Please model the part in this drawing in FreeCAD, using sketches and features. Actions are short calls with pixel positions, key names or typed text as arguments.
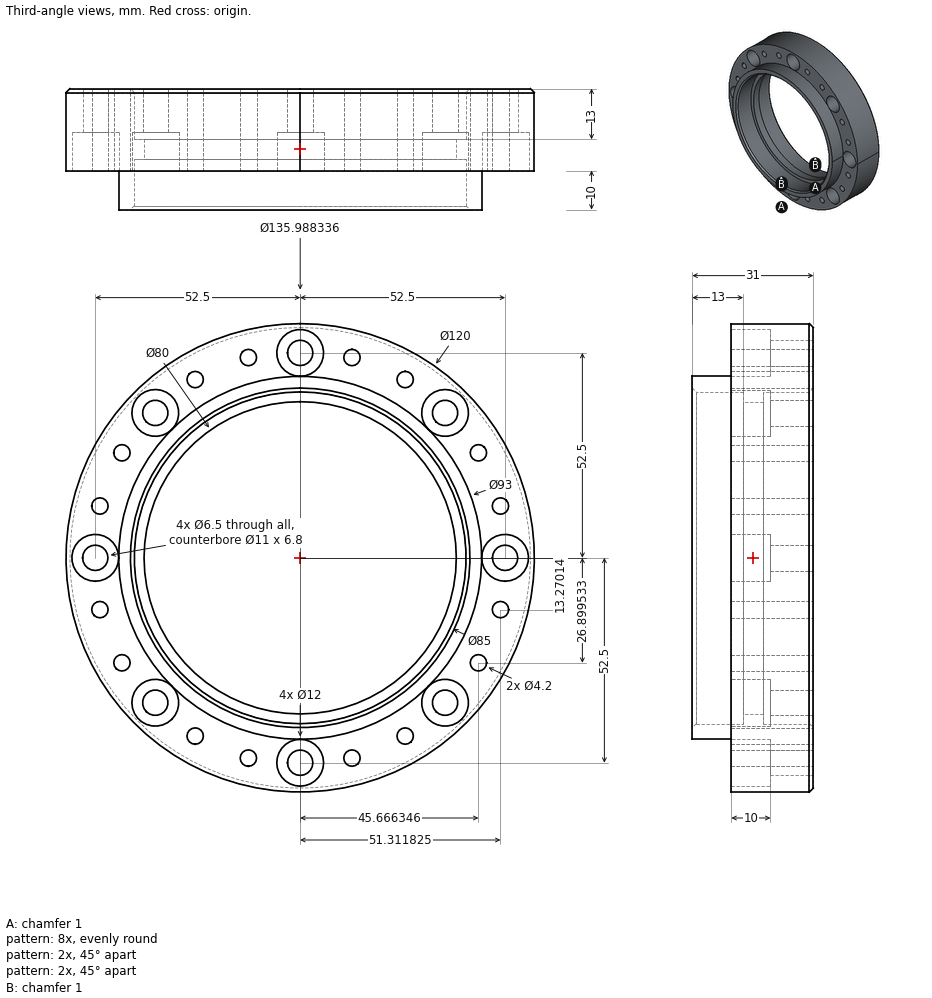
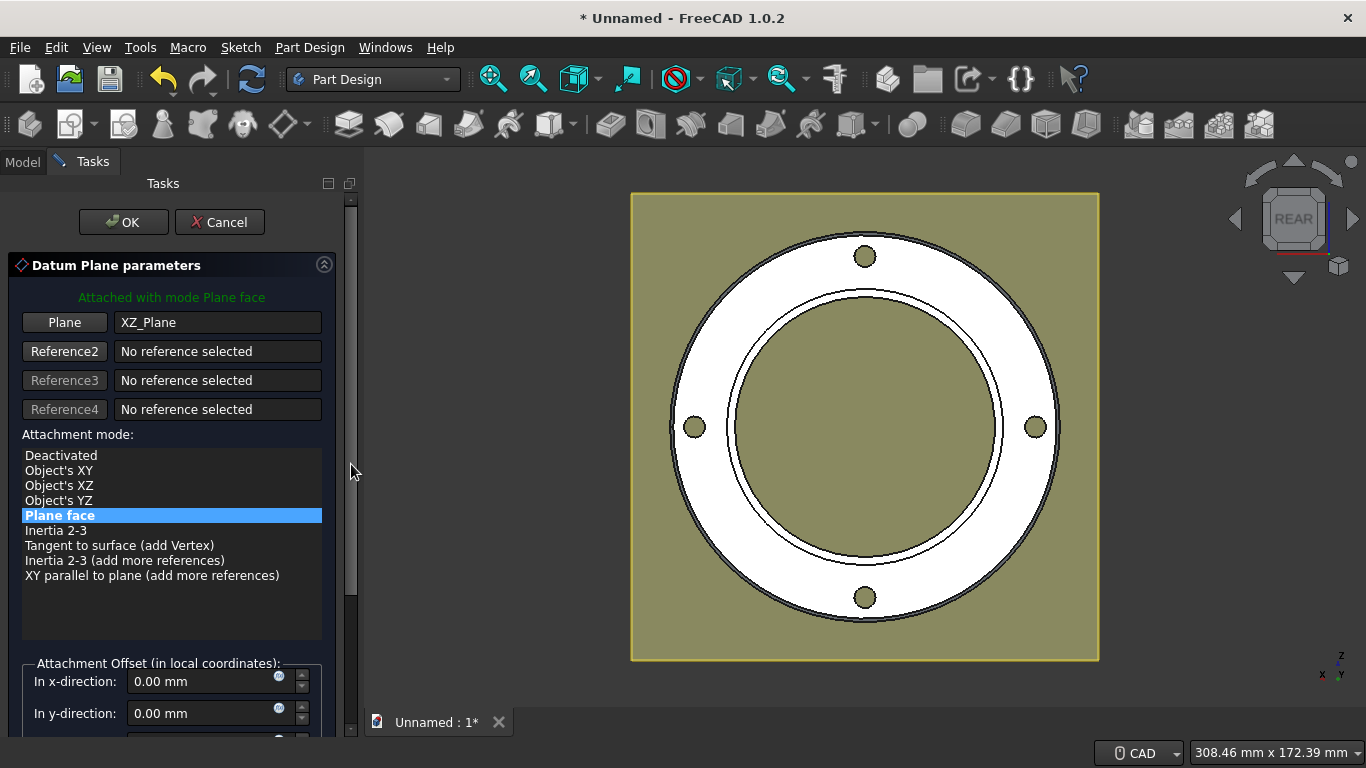
click(124, 222)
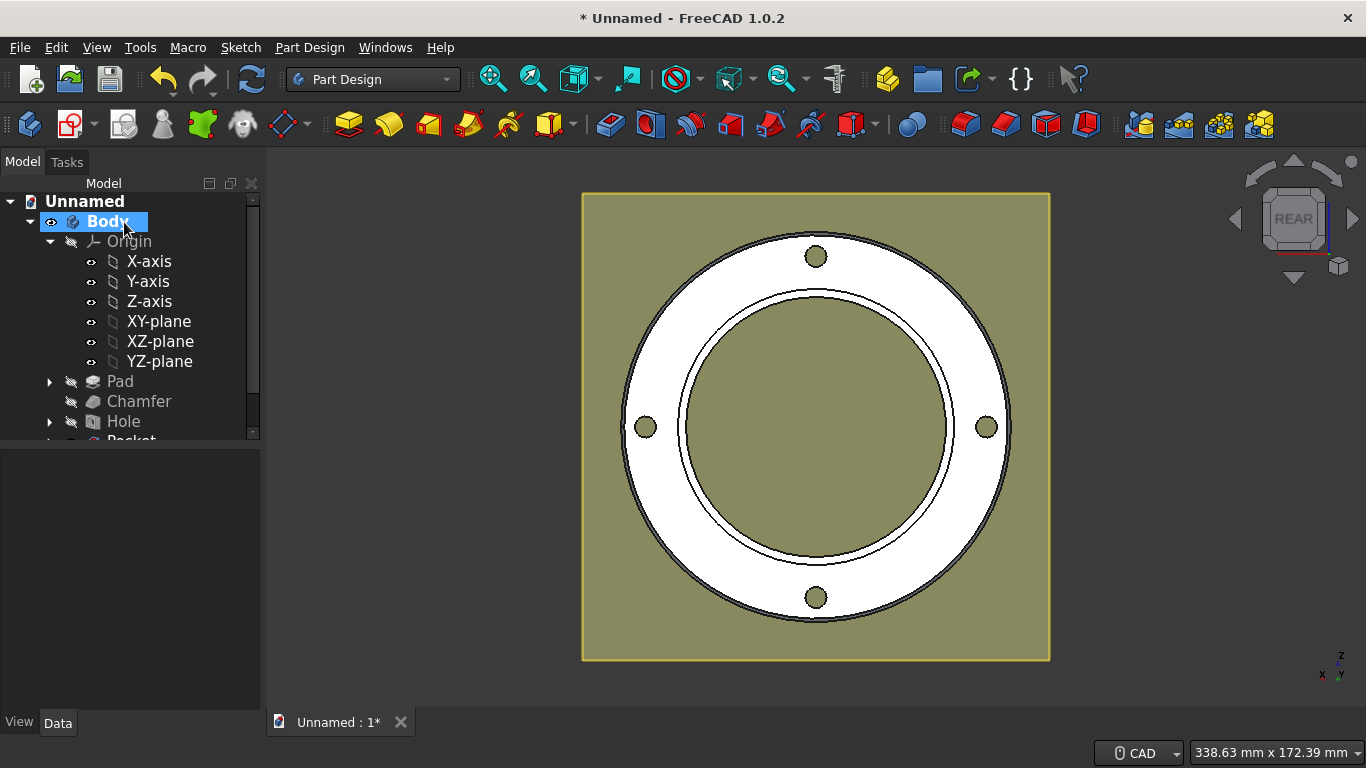
scroll(100, 317, down, 3)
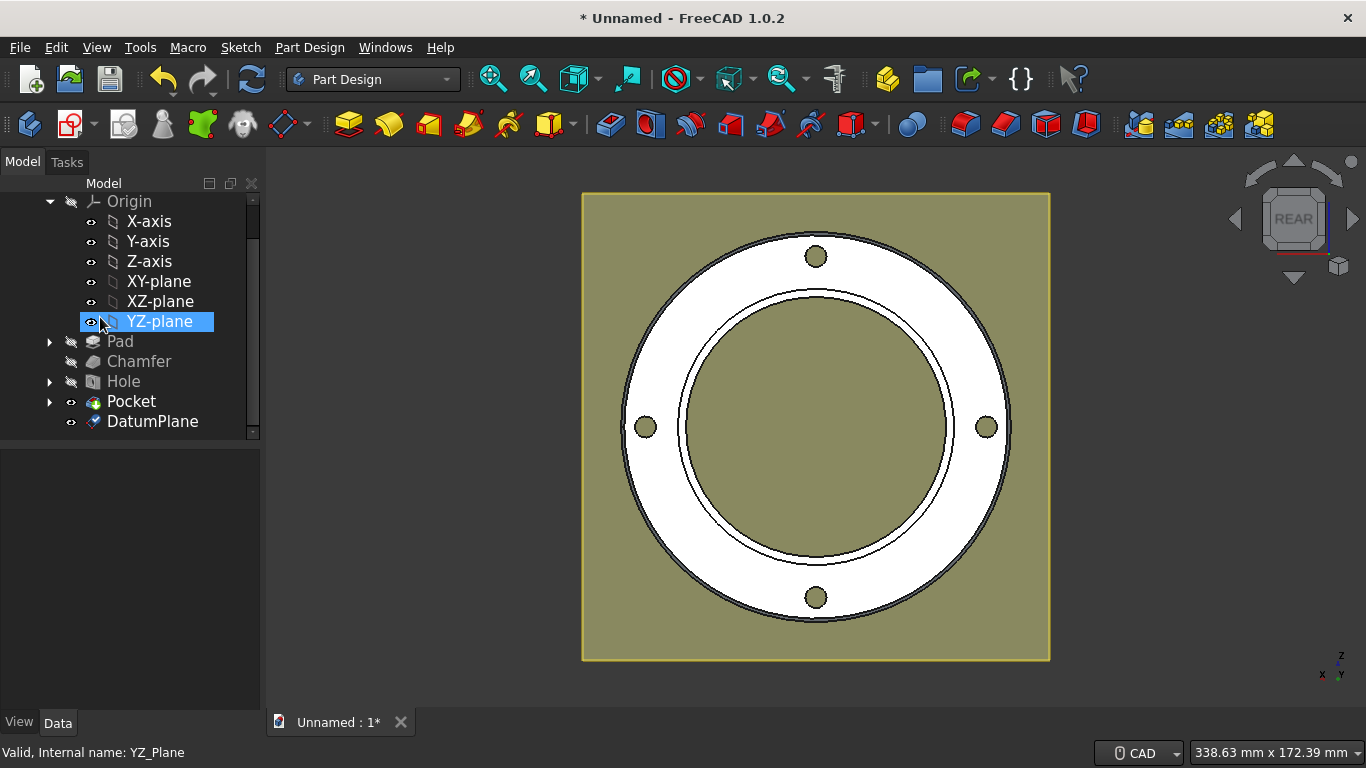
click(116, 422)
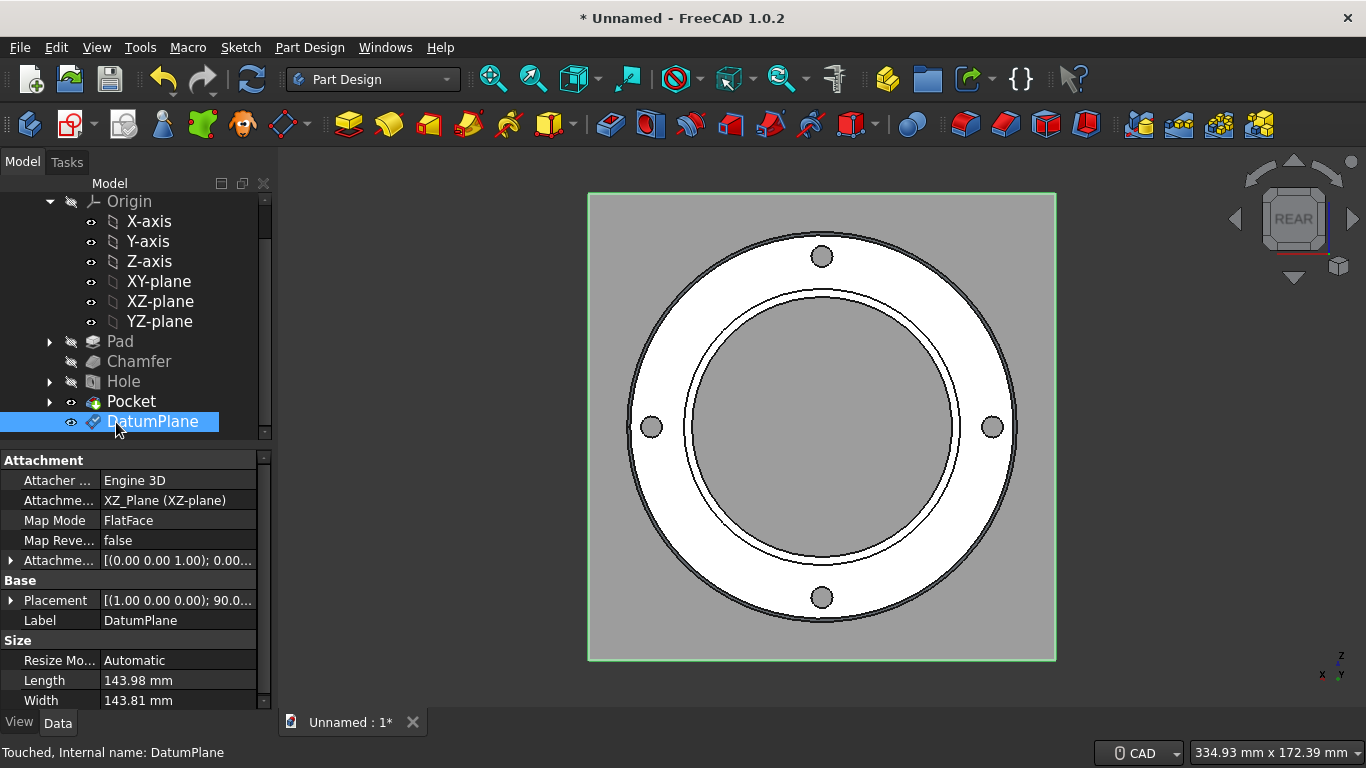
click(70, 124)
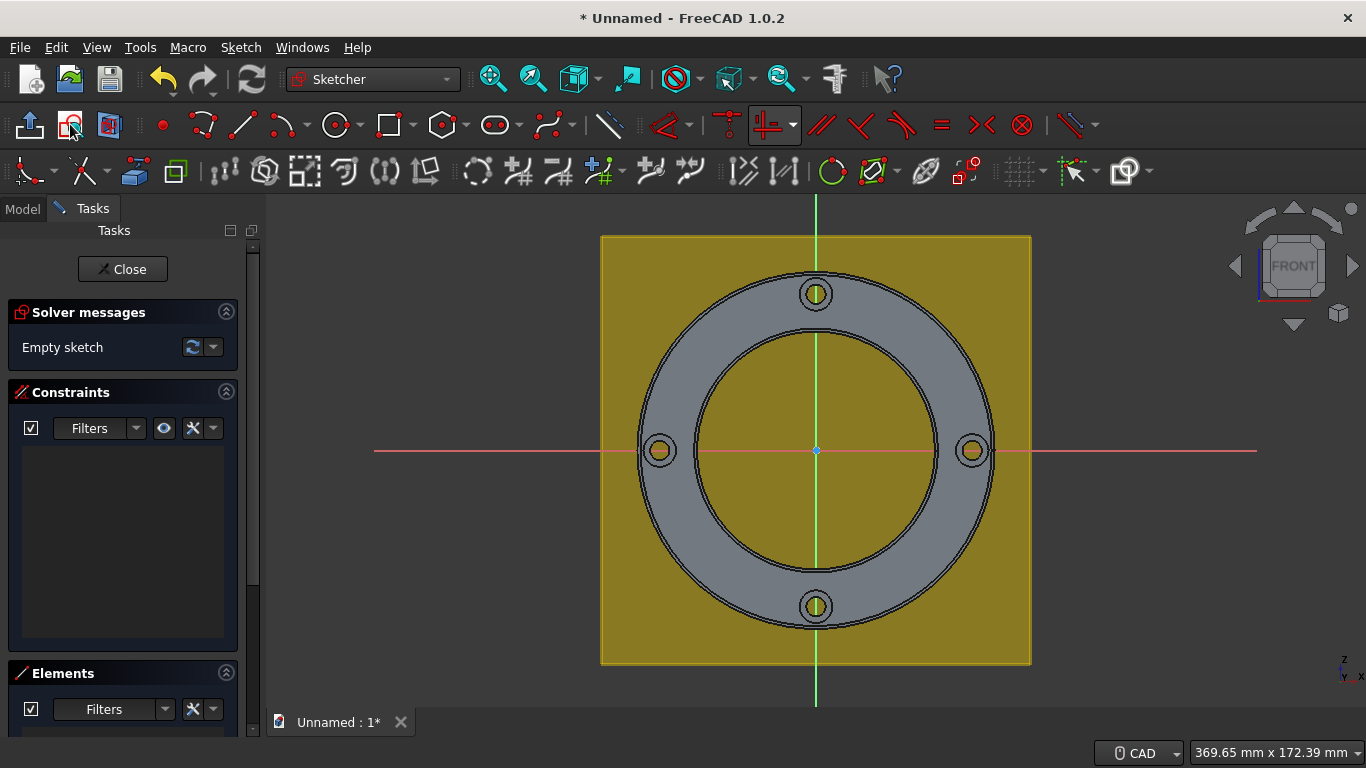
click(110, 126)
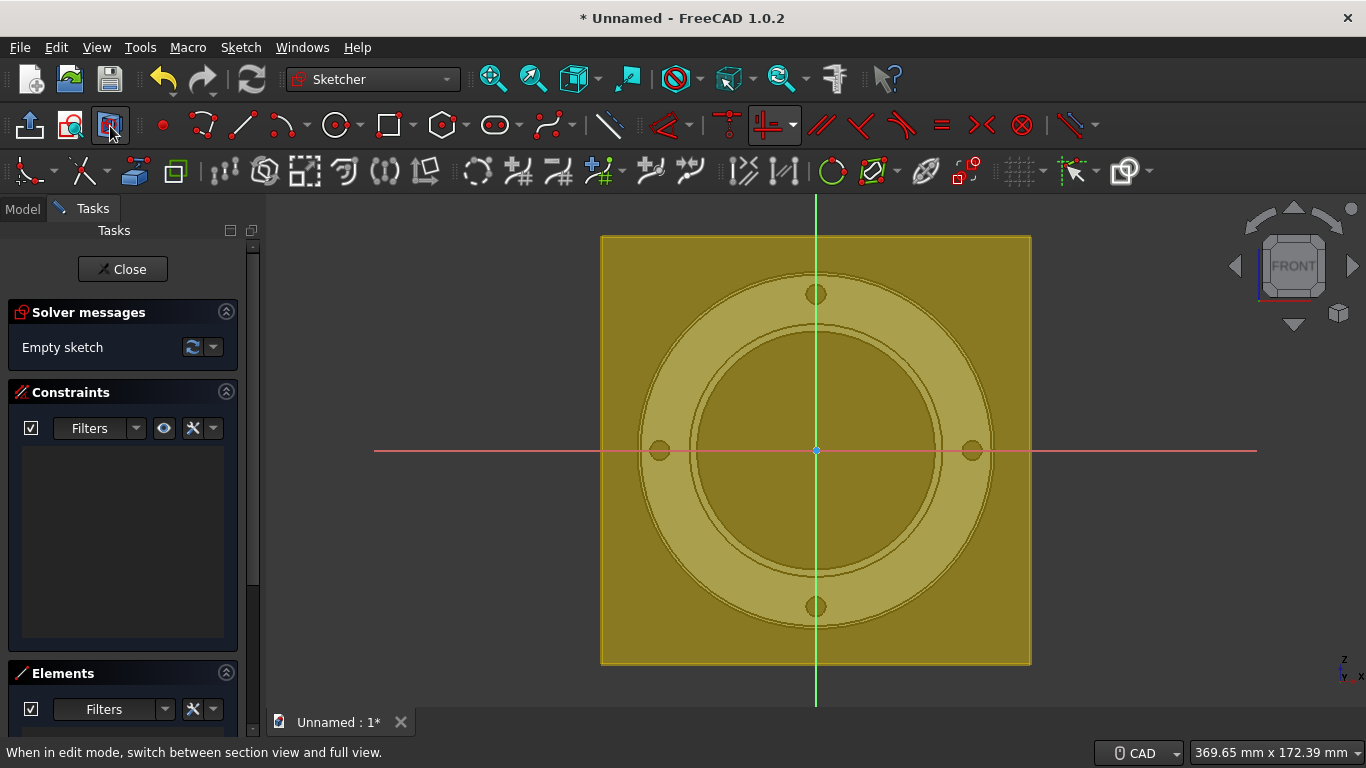
click(336, 126)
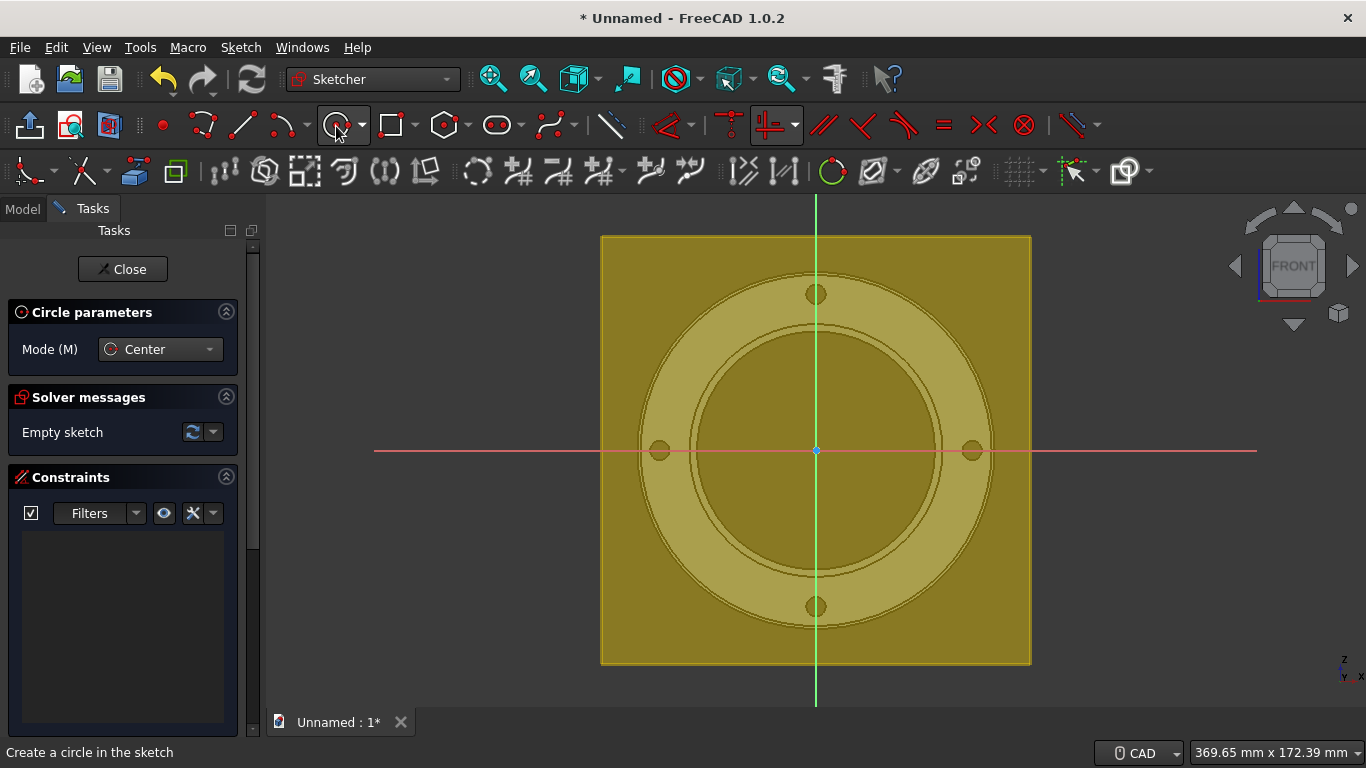
click(816, 451)
move(905, 361)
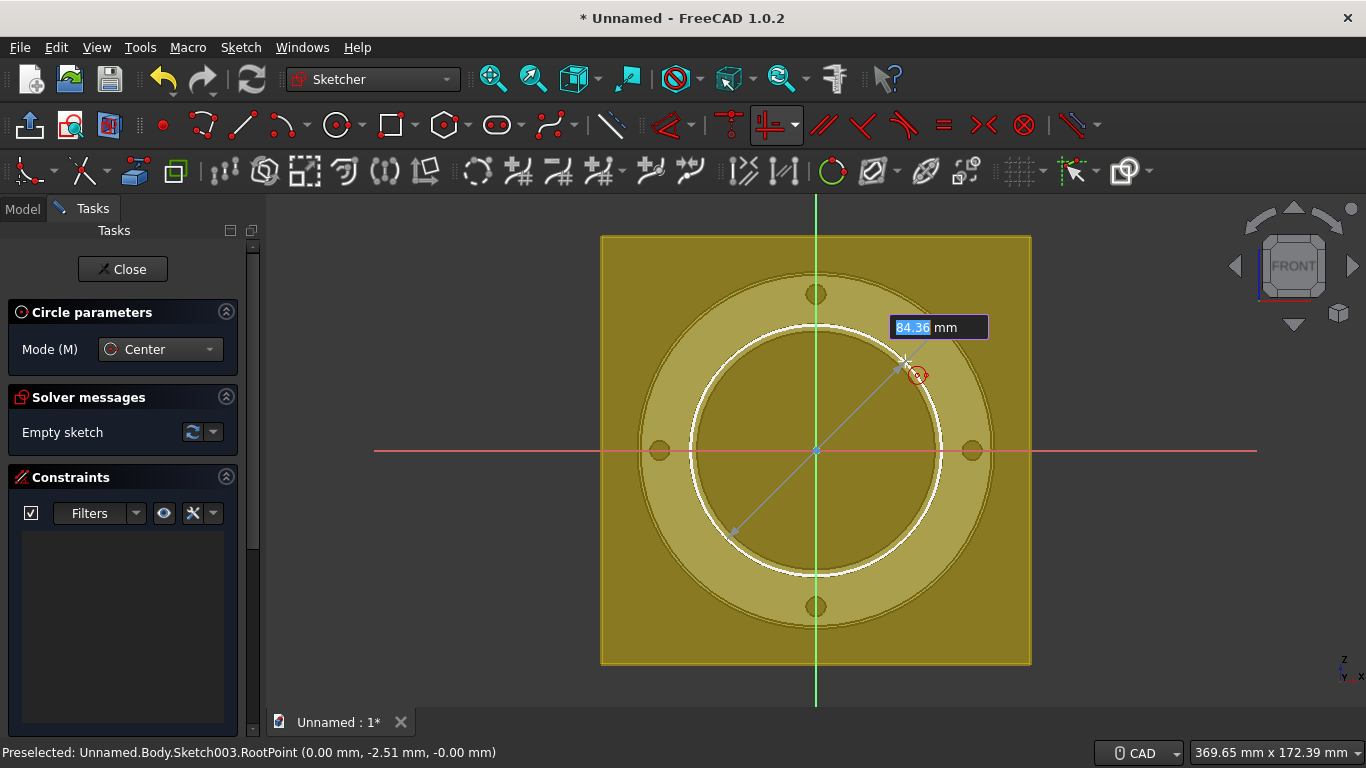
text(85)
key(Return)
key(Escape)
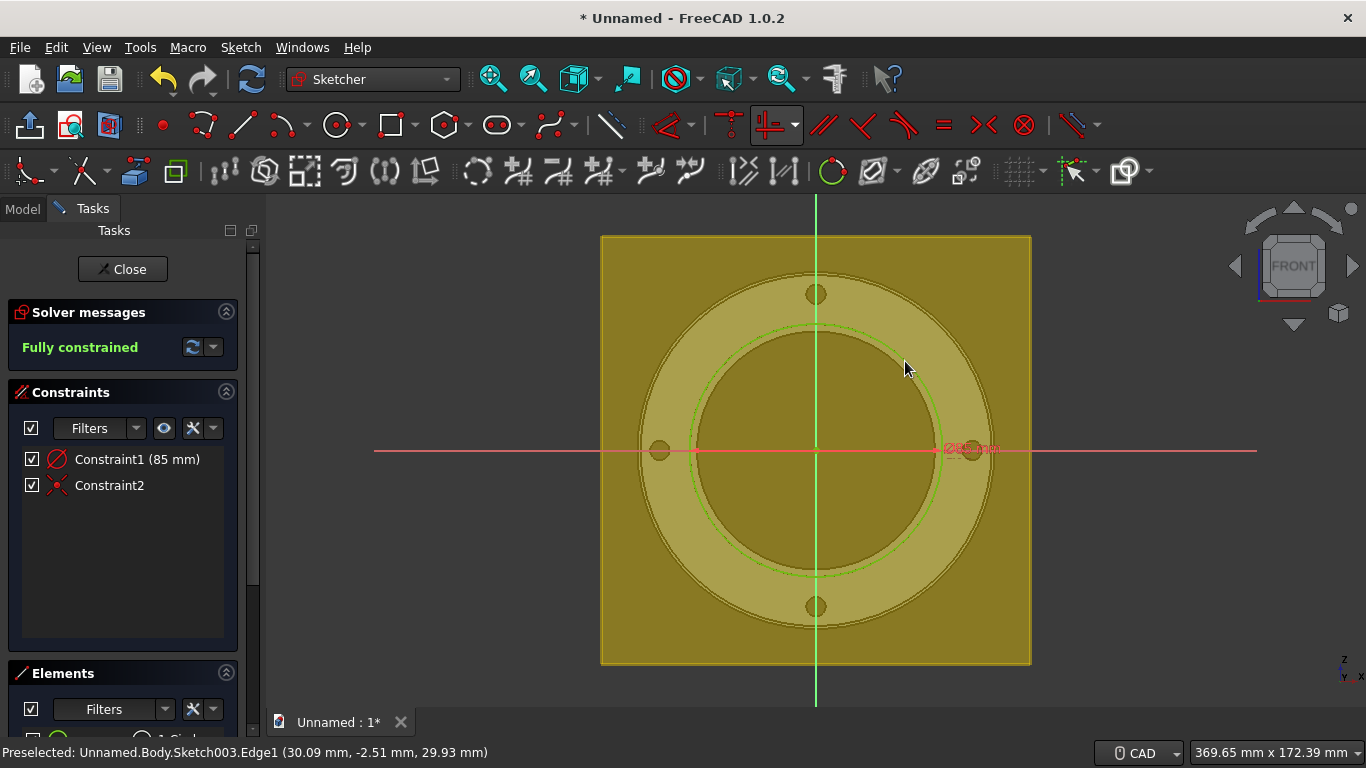
click(123, 269)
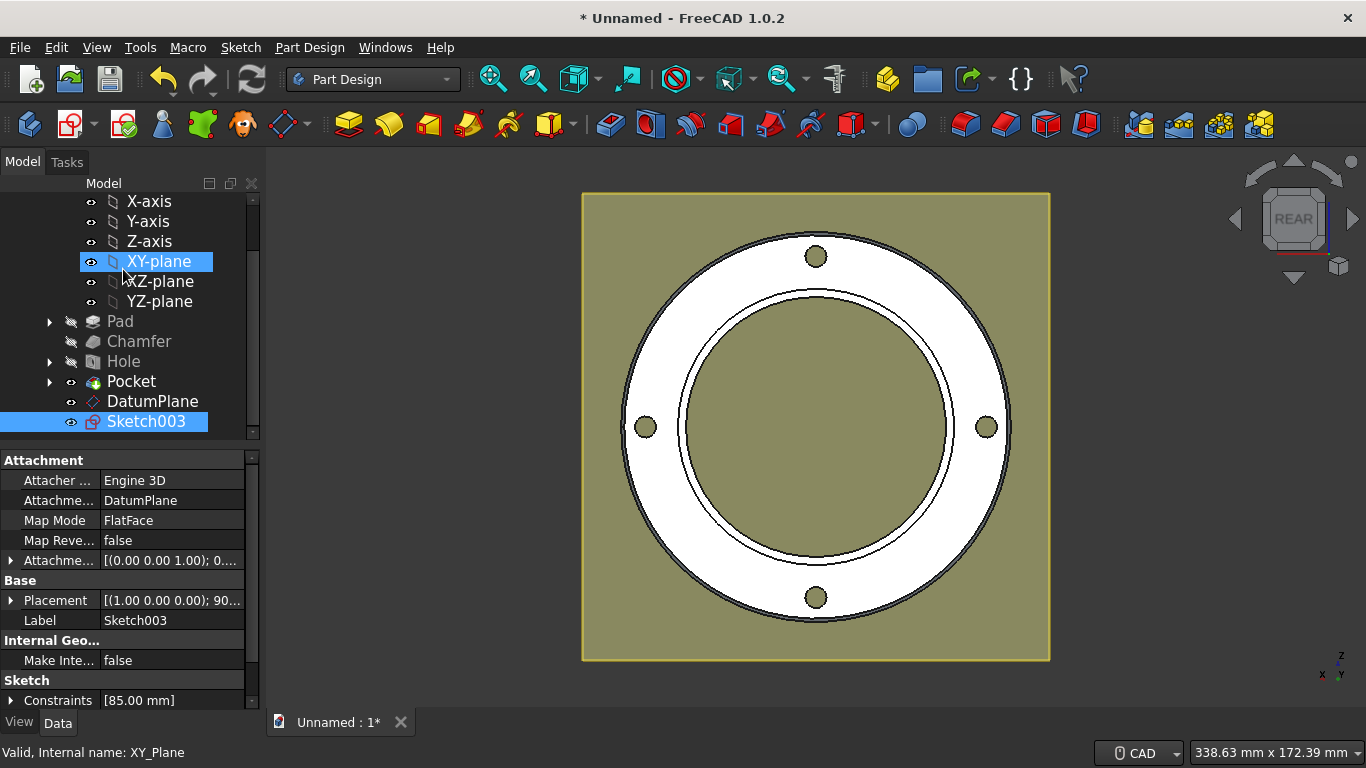
click(612, 124)